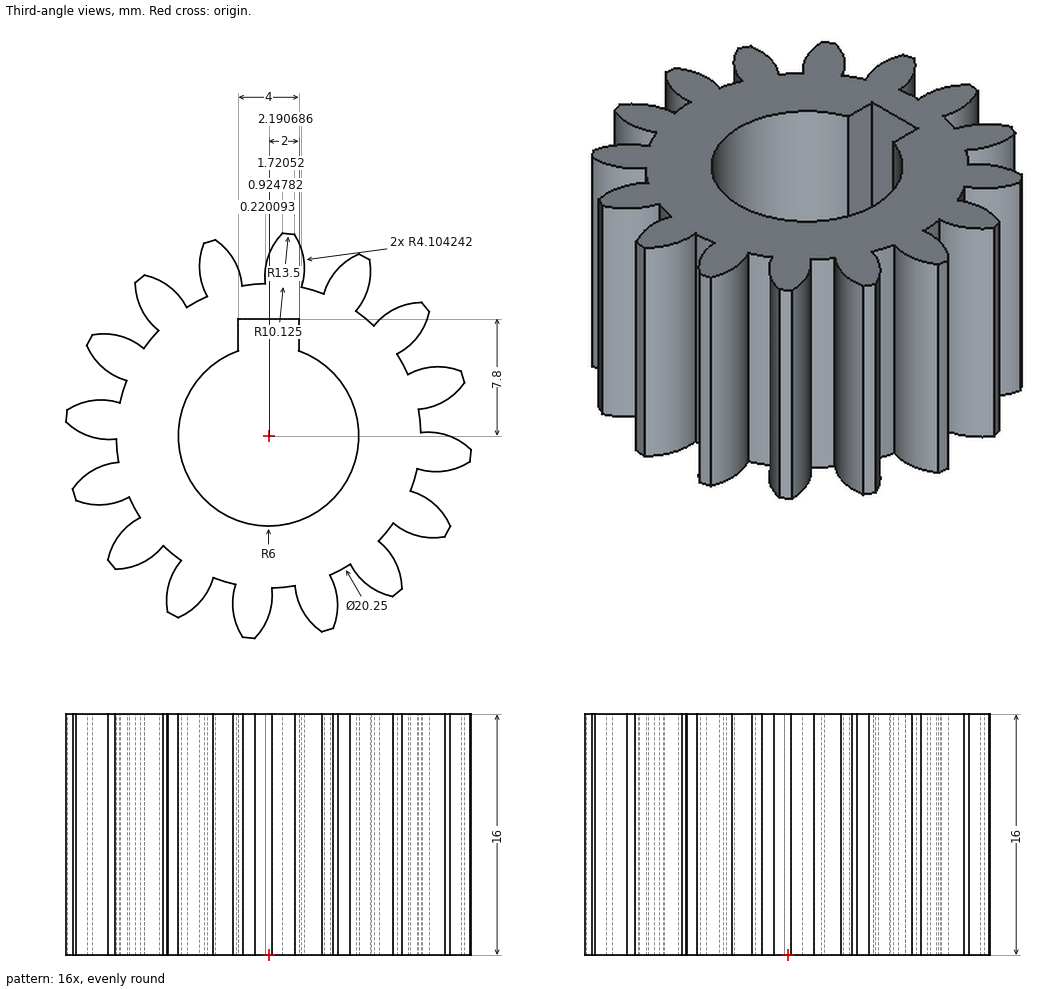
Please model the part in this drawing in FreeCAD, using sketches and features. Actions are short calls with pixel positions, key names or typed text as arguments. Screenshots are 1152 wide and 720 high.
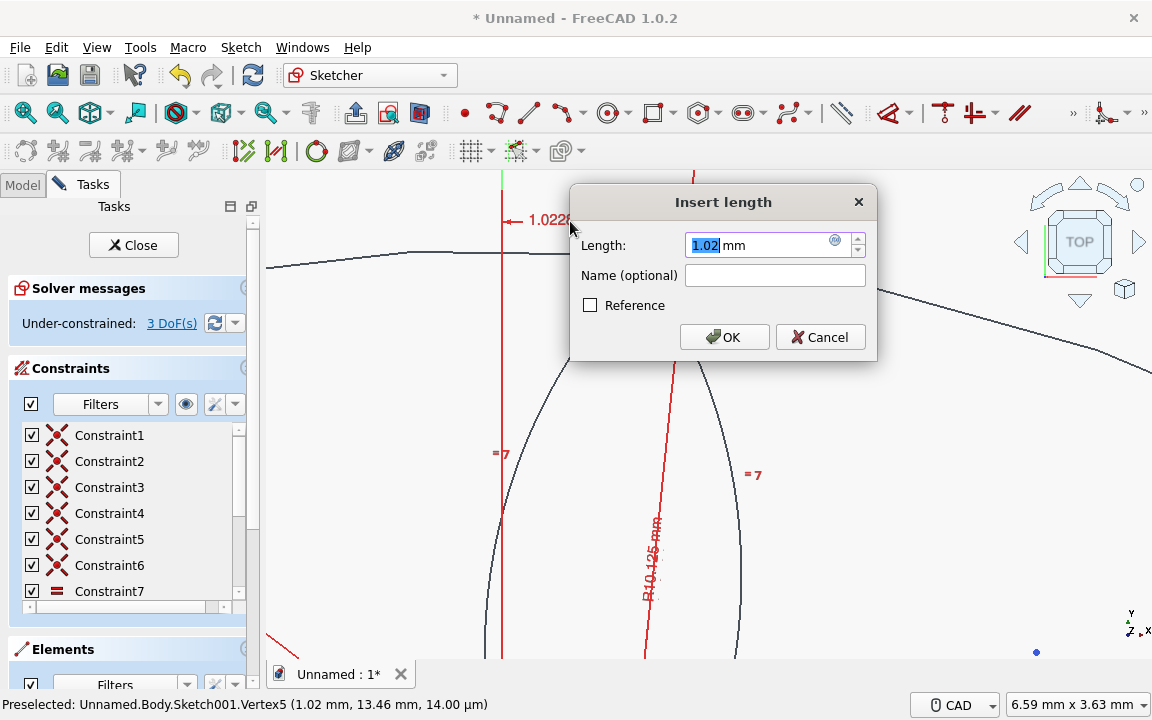
text(1.72052)
key(Return)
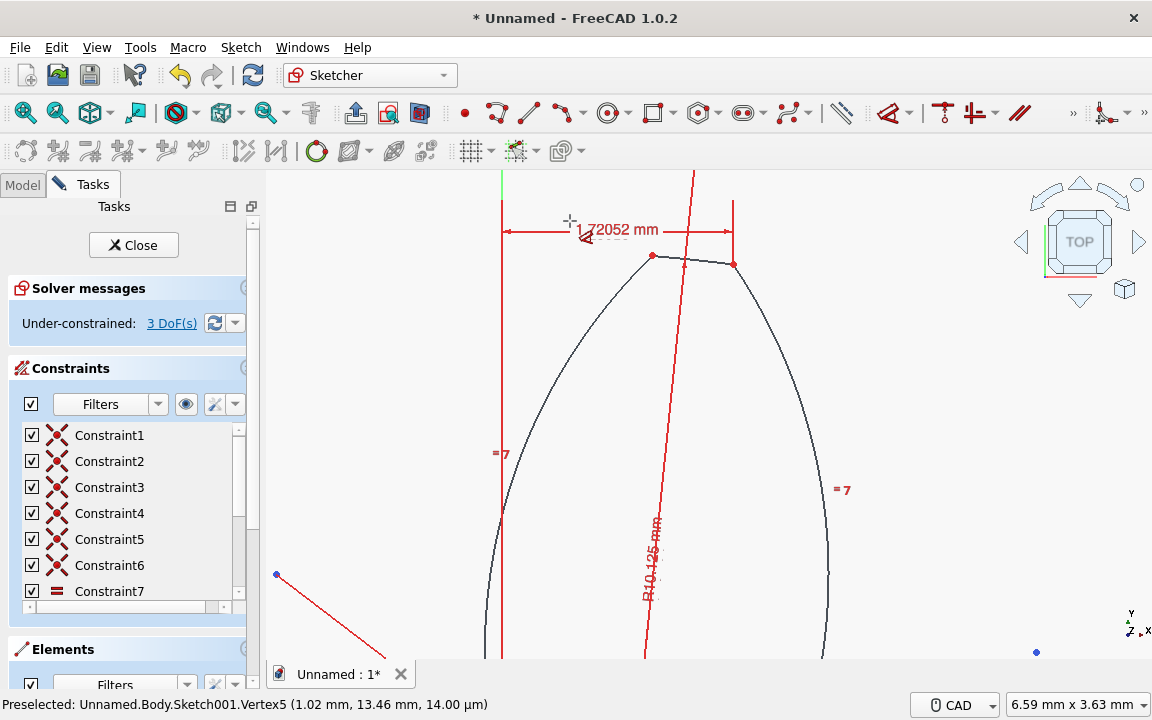
scroll(631, 251, down, 2)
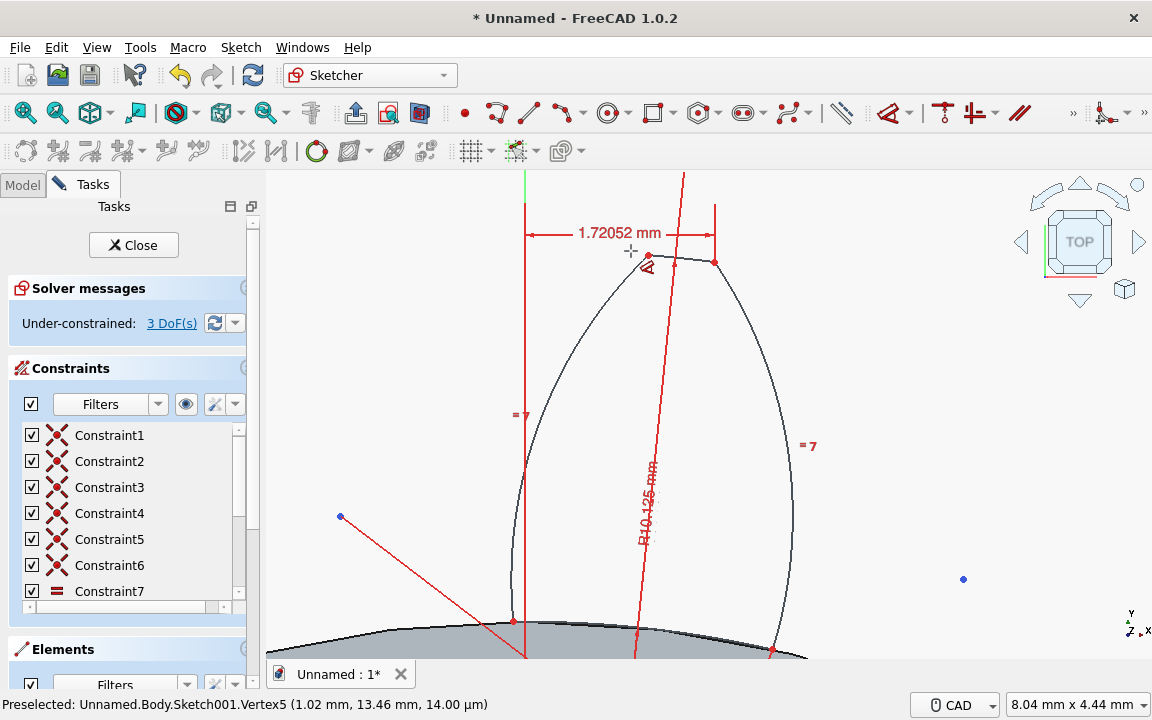
click(747, 577)
click(646, 543)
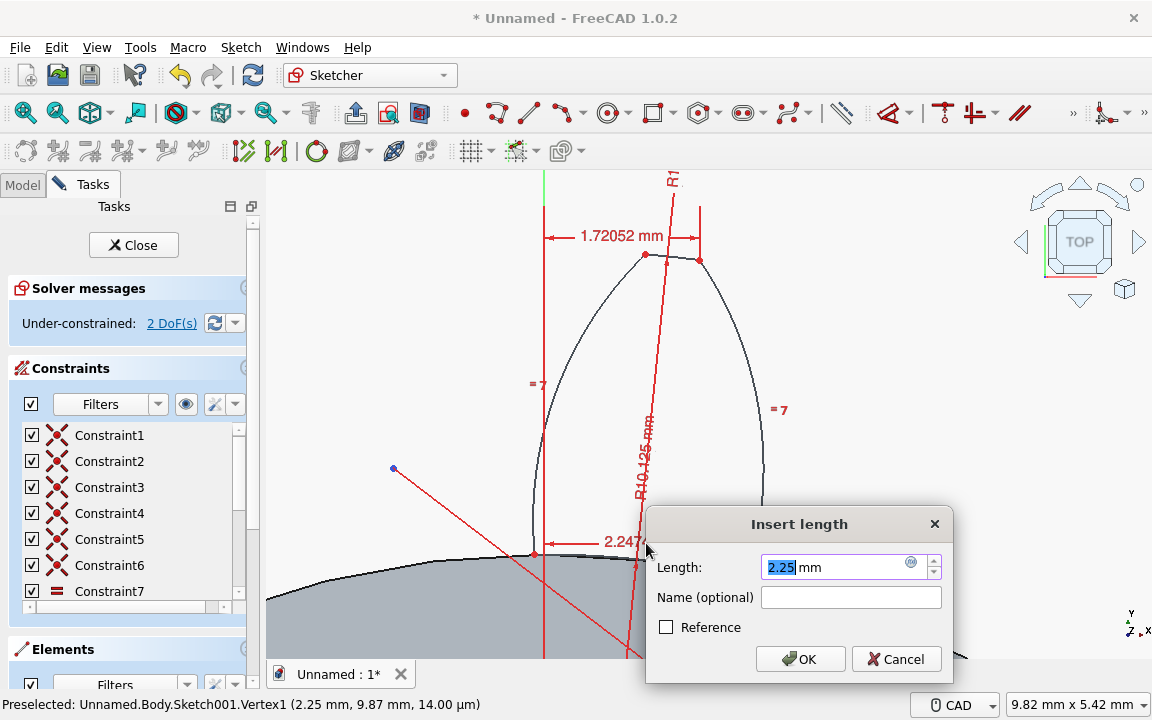
text(2.190686)
key(Return)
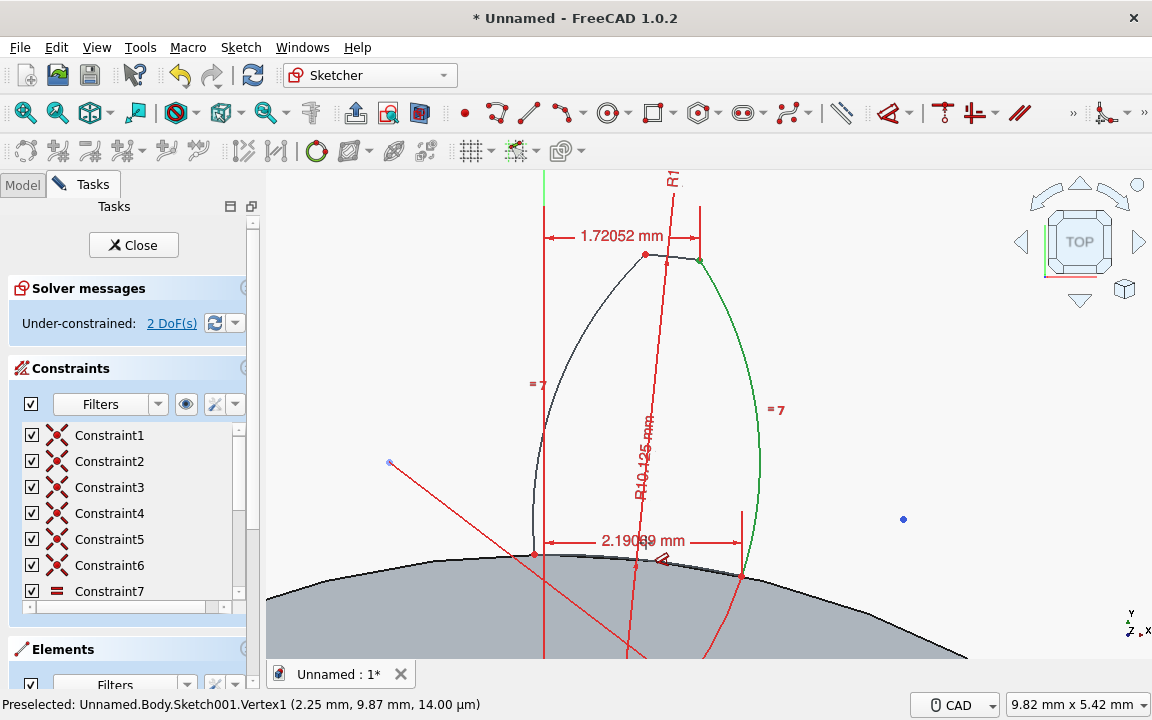
scroll(535, 555, up, 4)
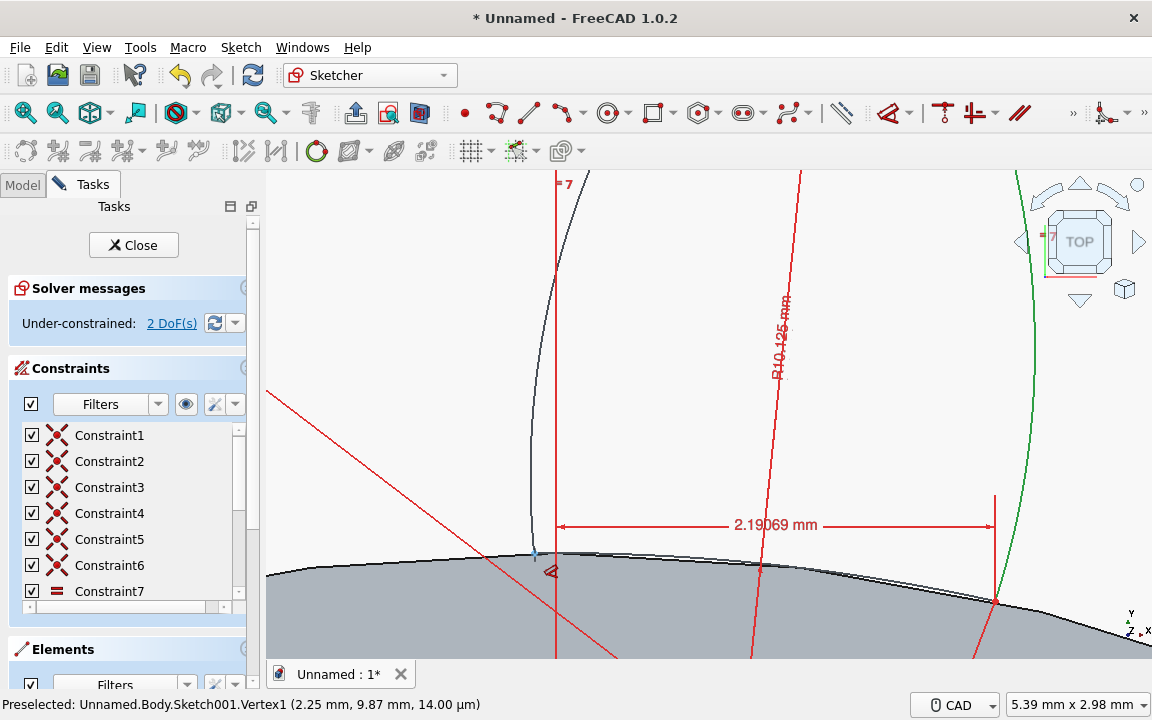
click(534, 553)
click(545, 519)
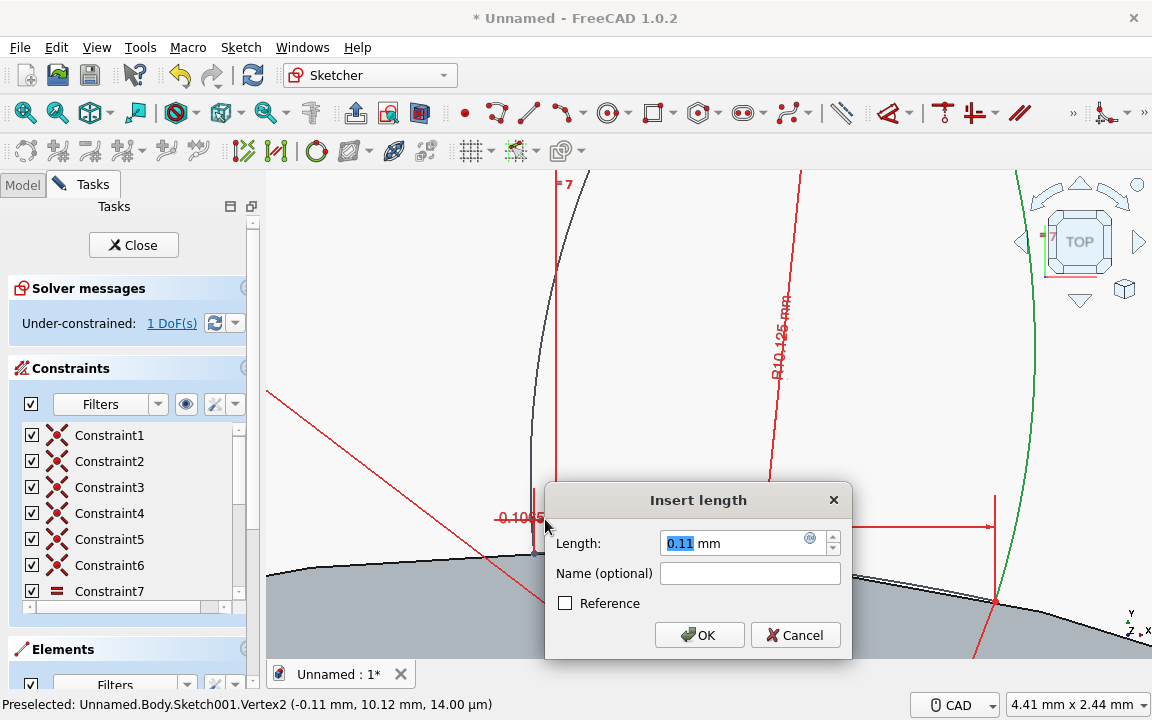
text(0.220093)
key(Return)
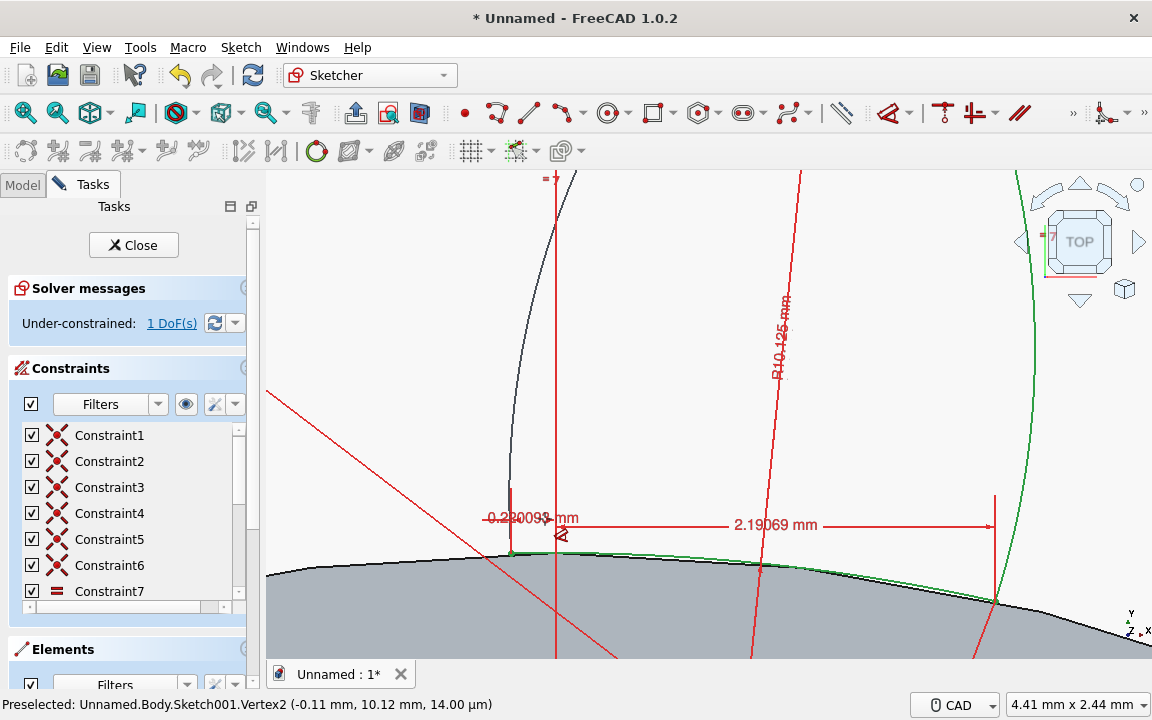
scroll(535, 556, down, 4)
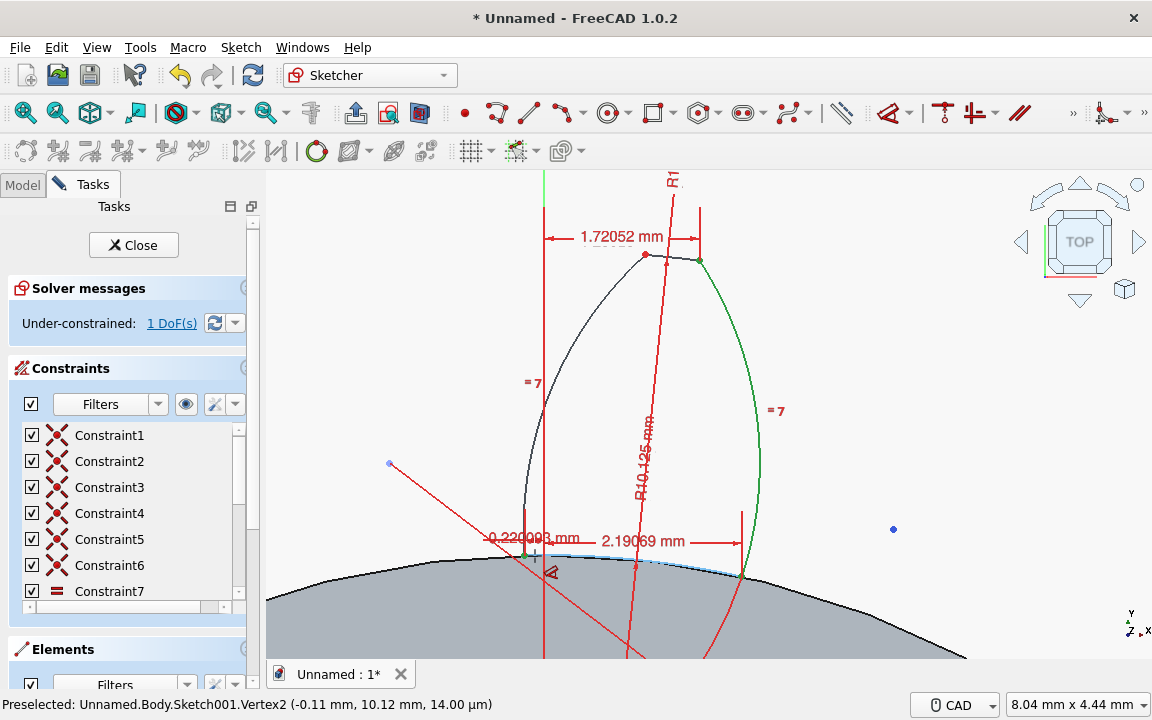
click(645, 255)
click(595, 221)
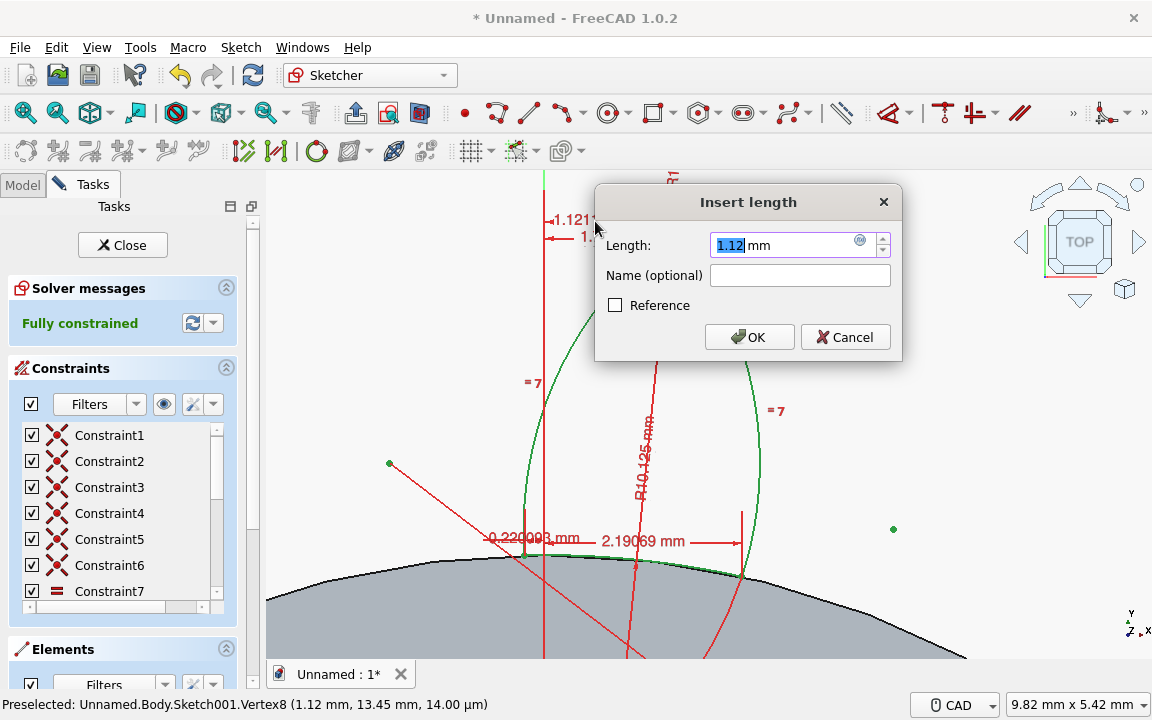
text(0.924782)
key(Return)
key(Escape)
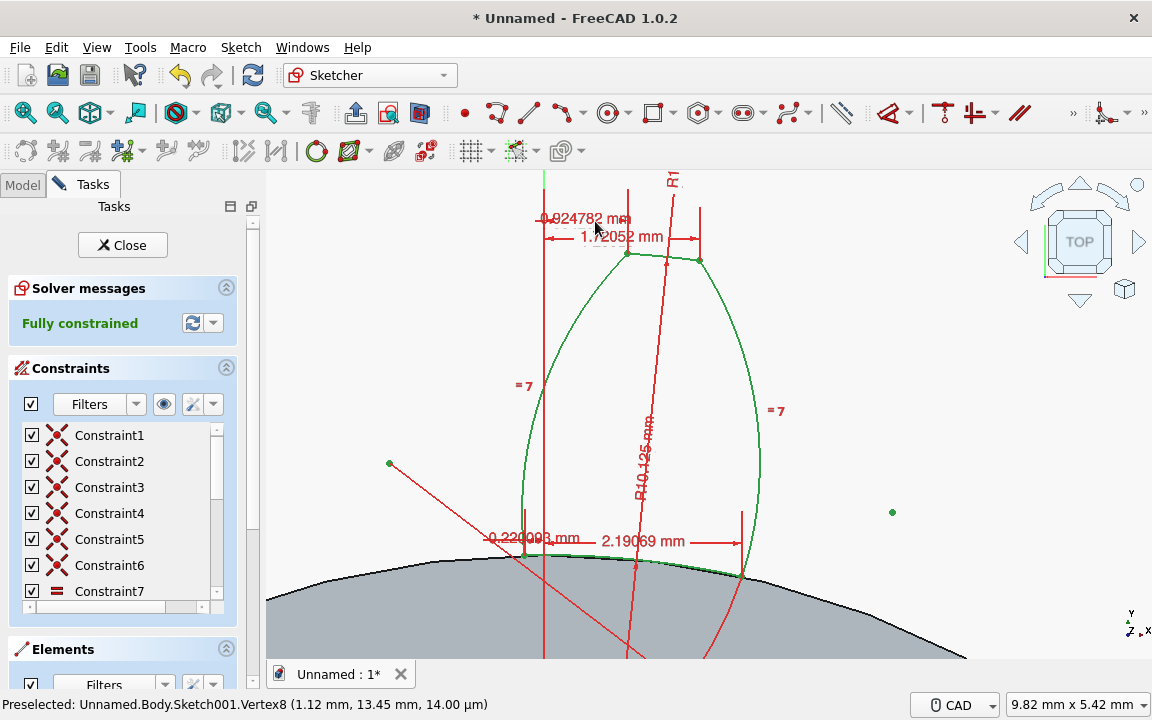
click(123, 245)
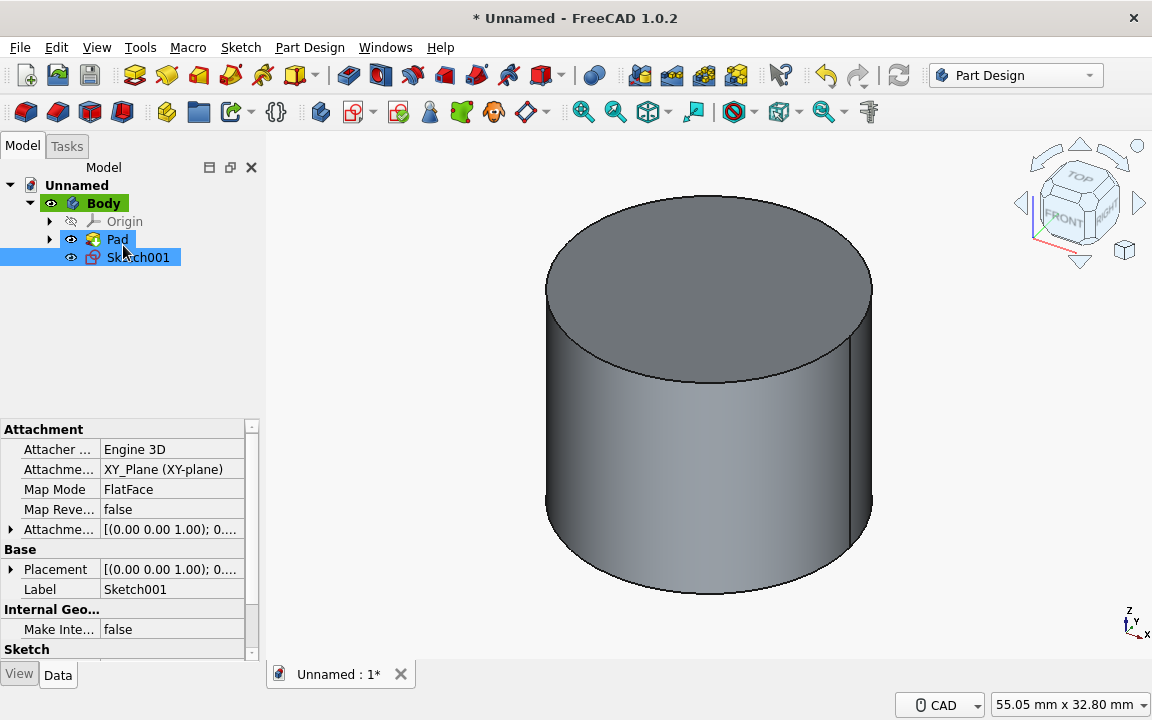
click(136, 76)